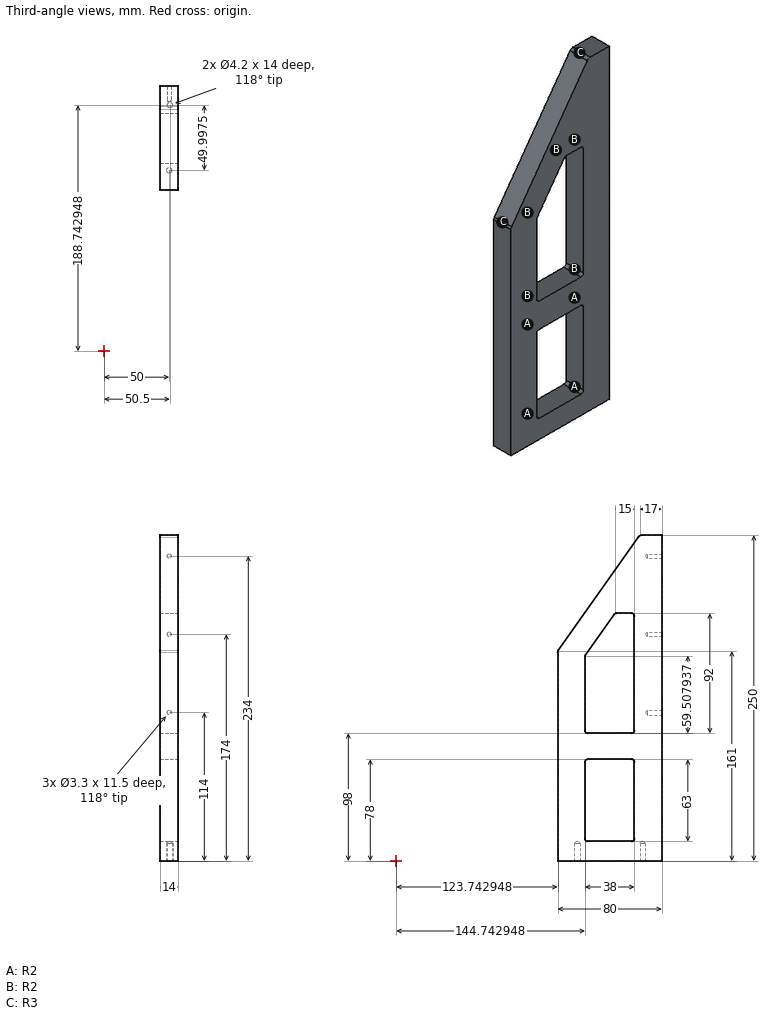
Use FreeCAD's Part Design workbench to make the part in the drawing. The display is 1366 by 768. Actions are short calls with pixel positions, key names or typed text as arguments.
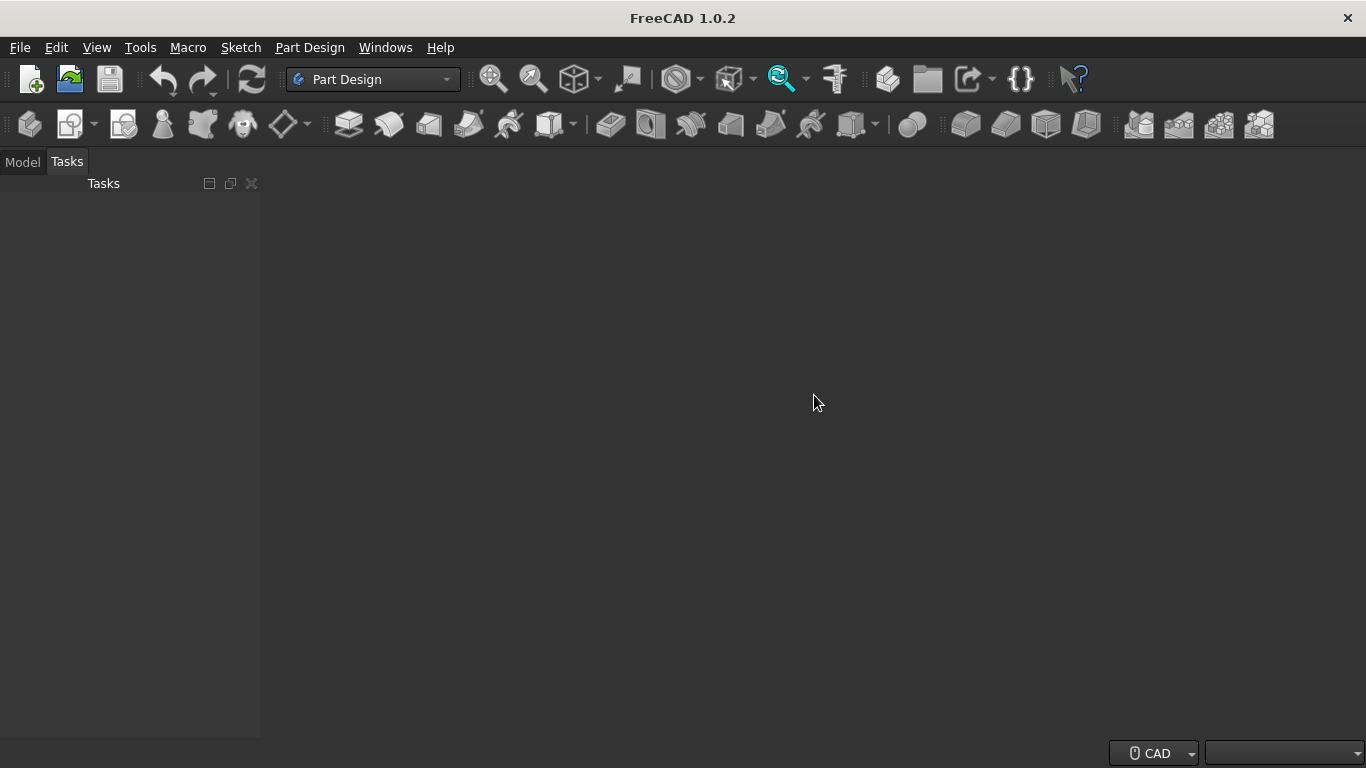
click(30, 80)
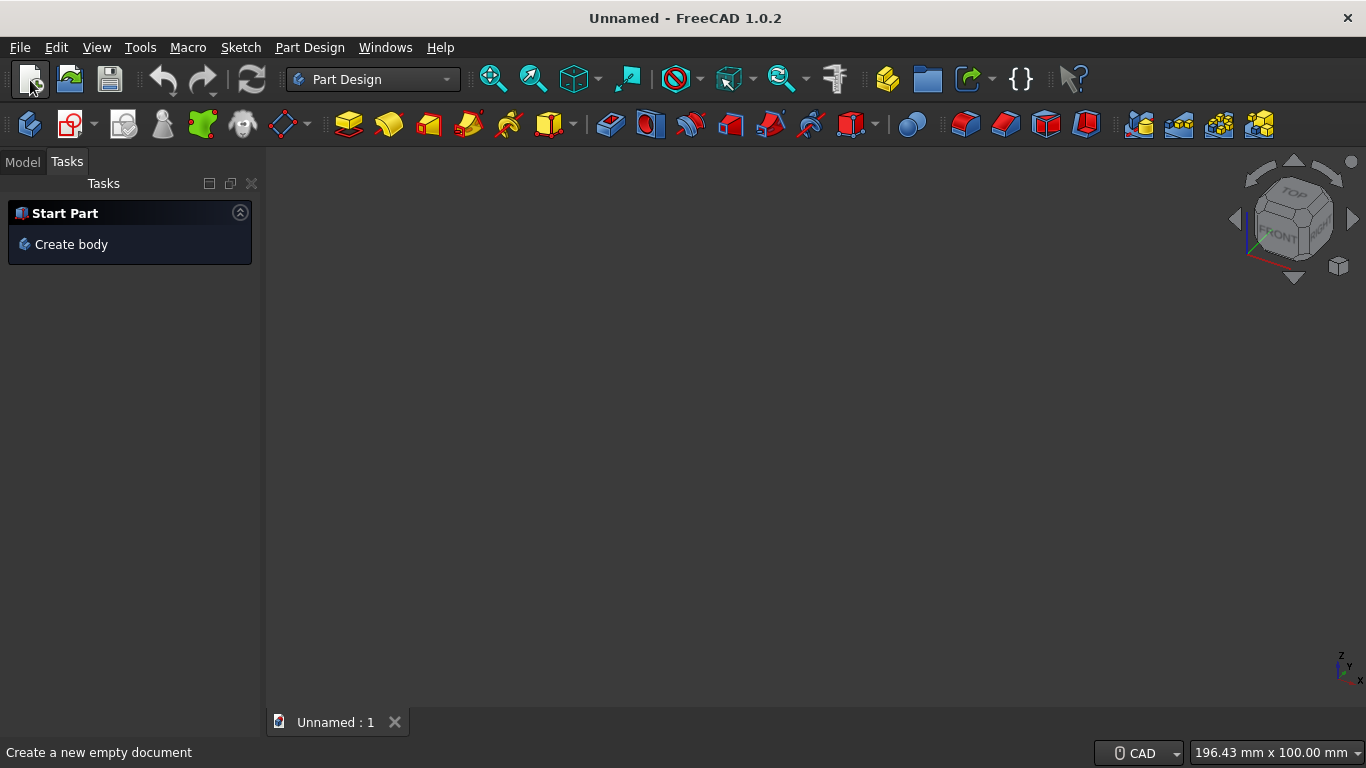
click(30, 124)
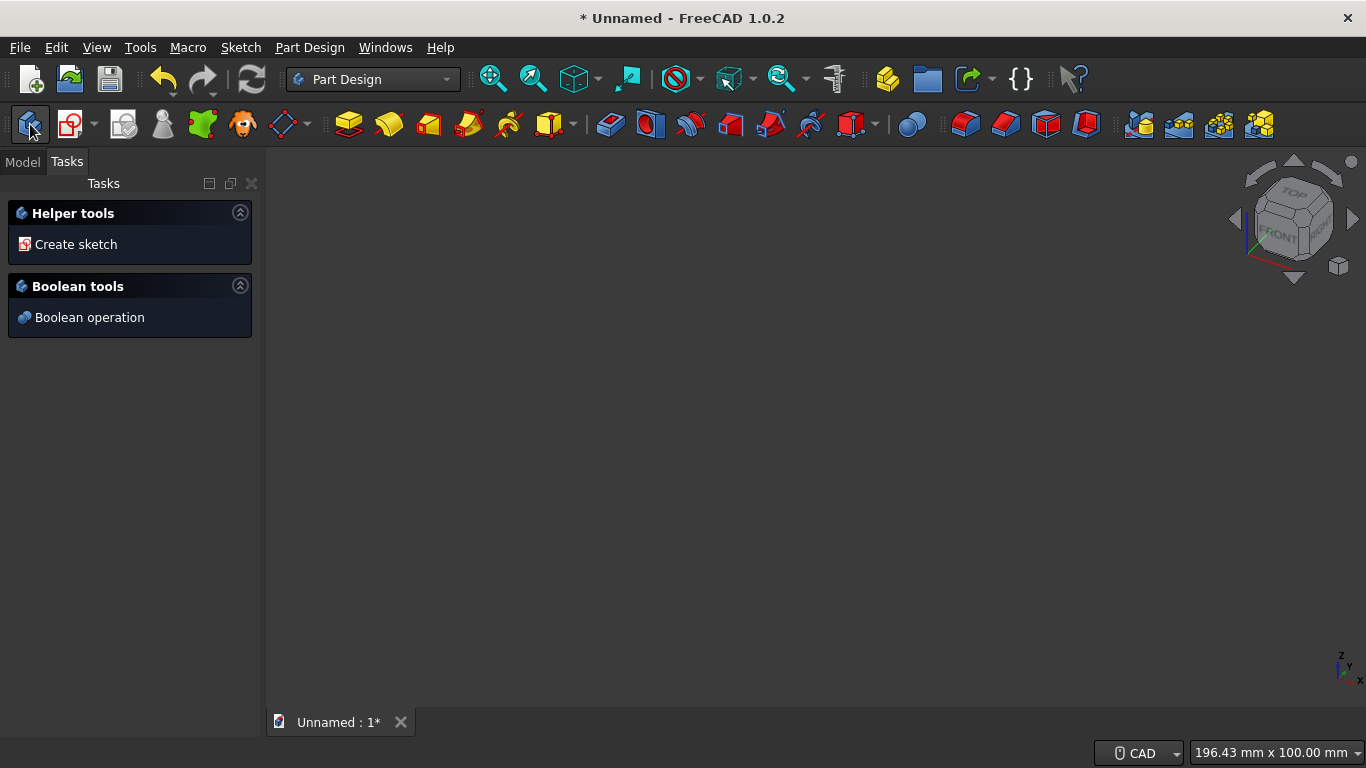
click(23, 161)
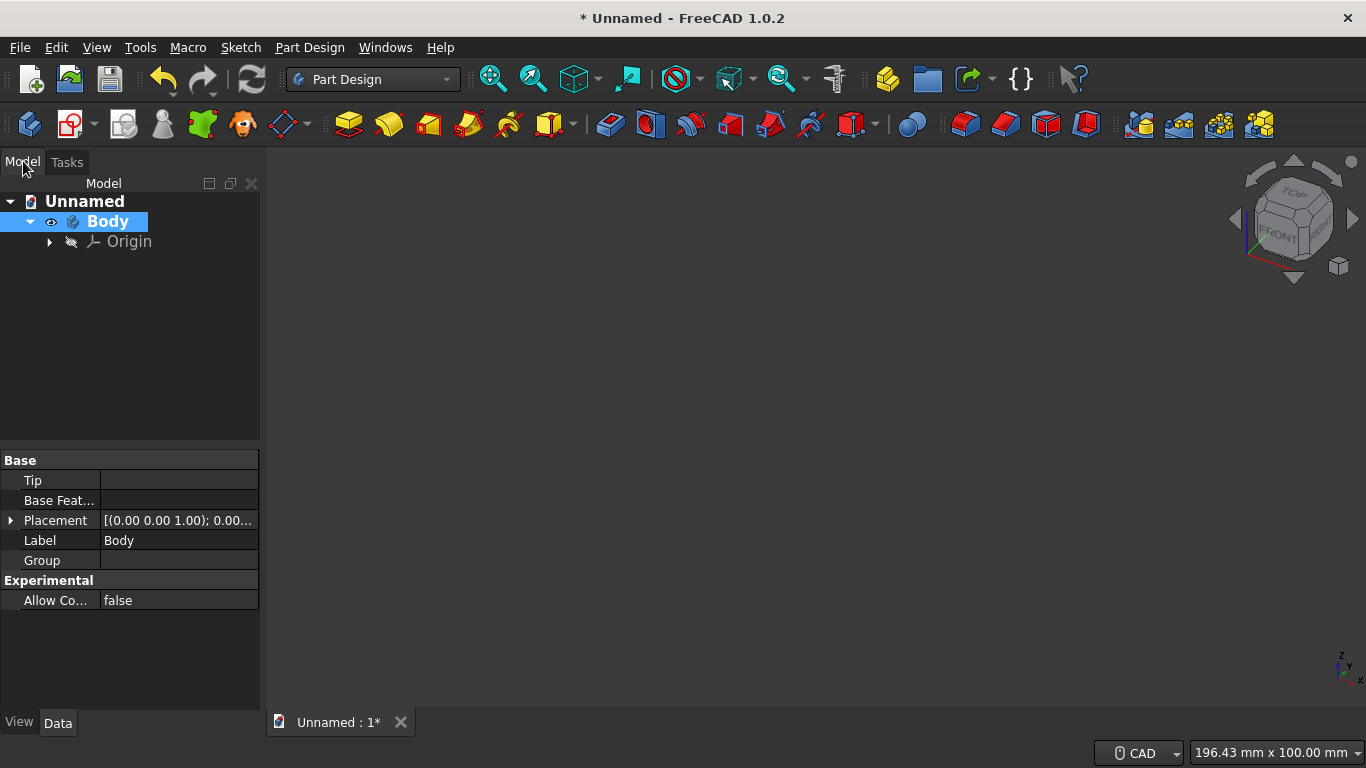
click(50, 242)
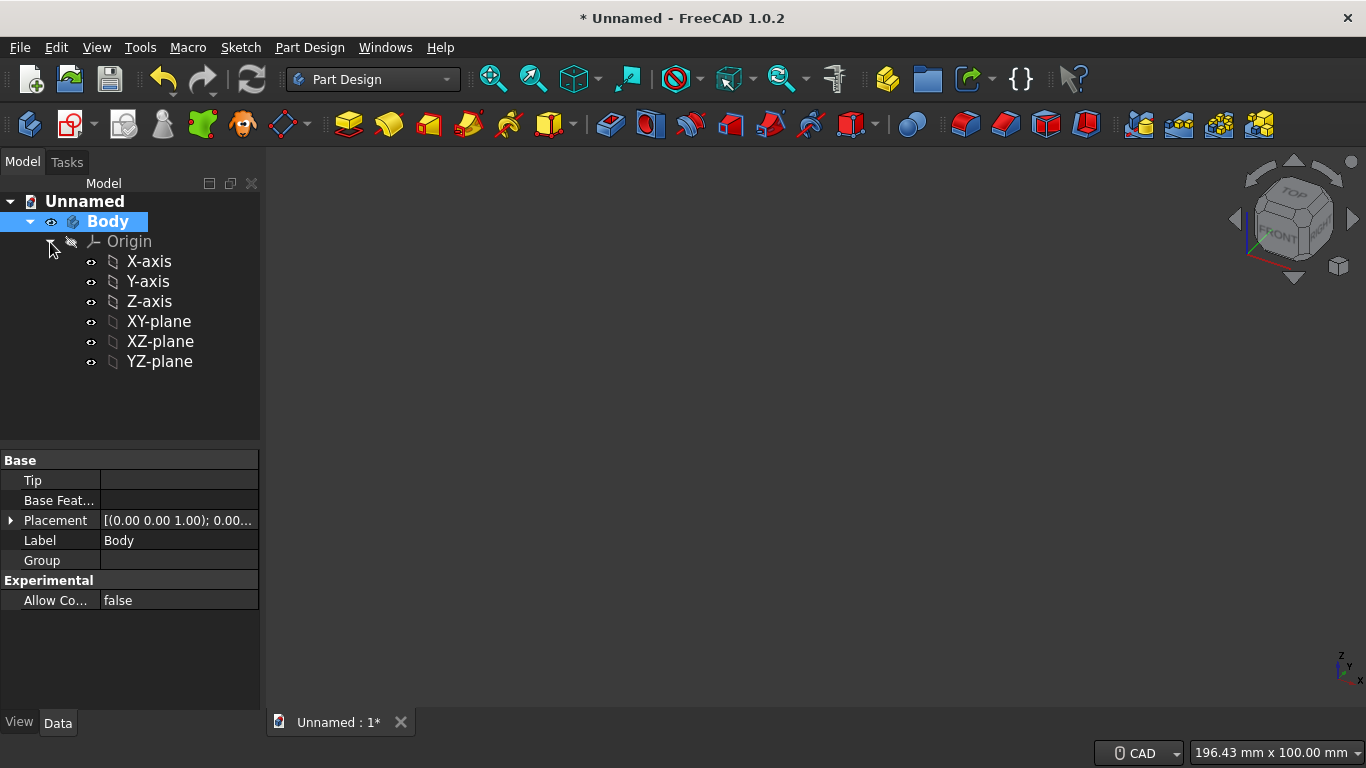
click(136, 362)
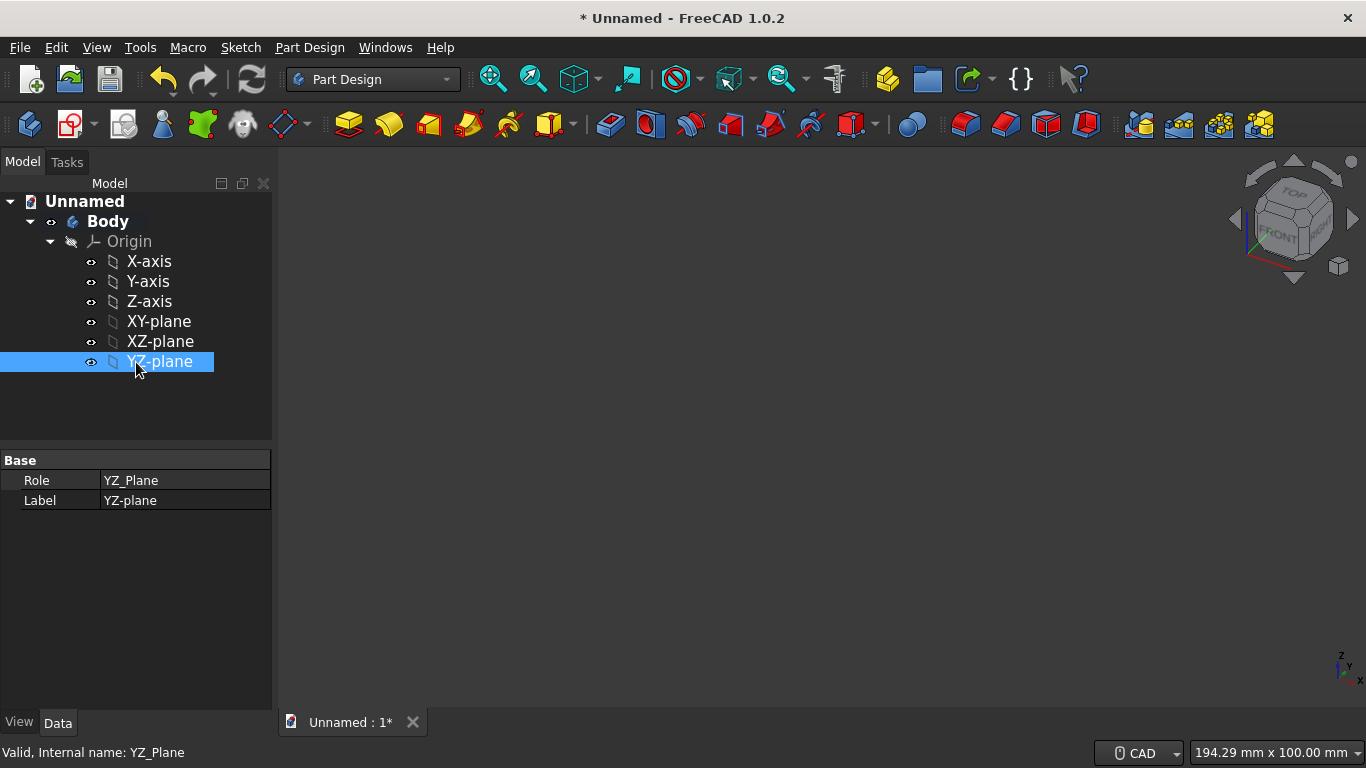
click(284, 124)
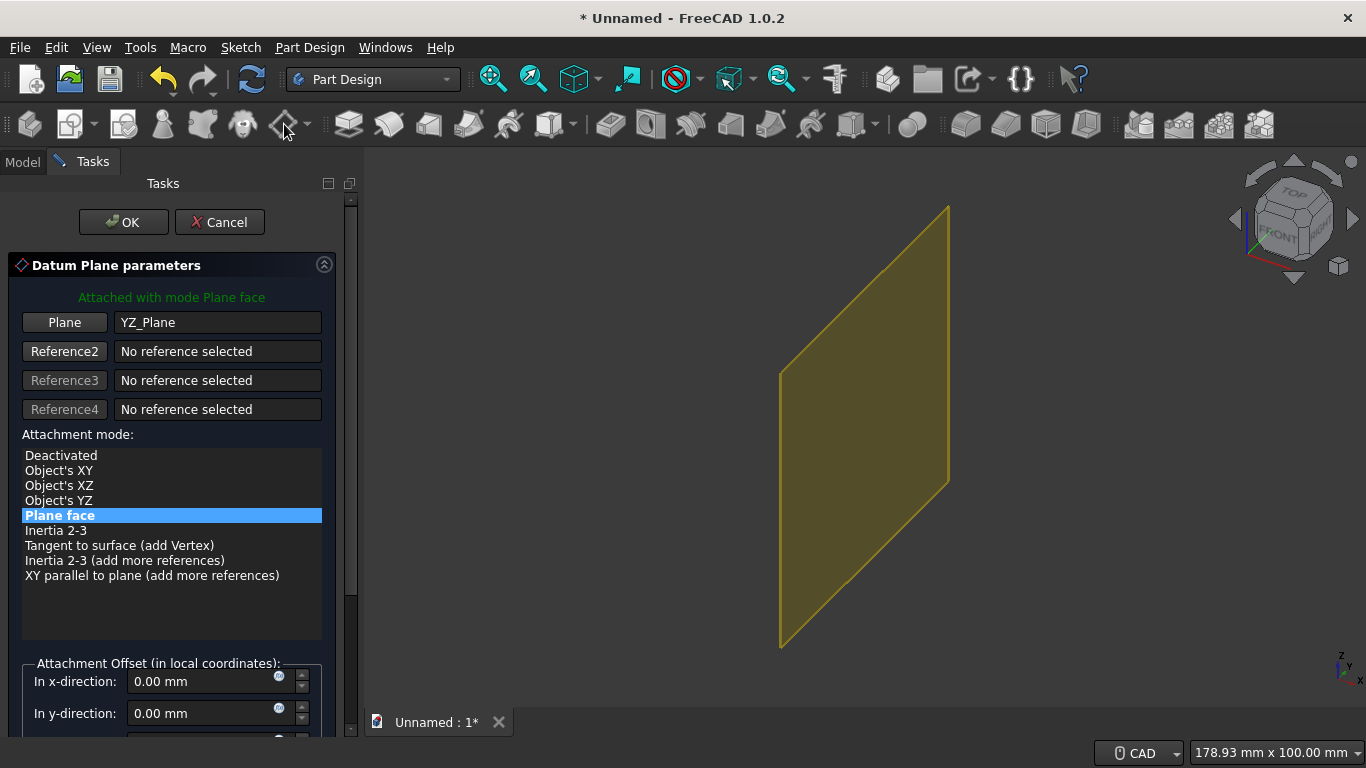
scroll(351, 464, down, 2)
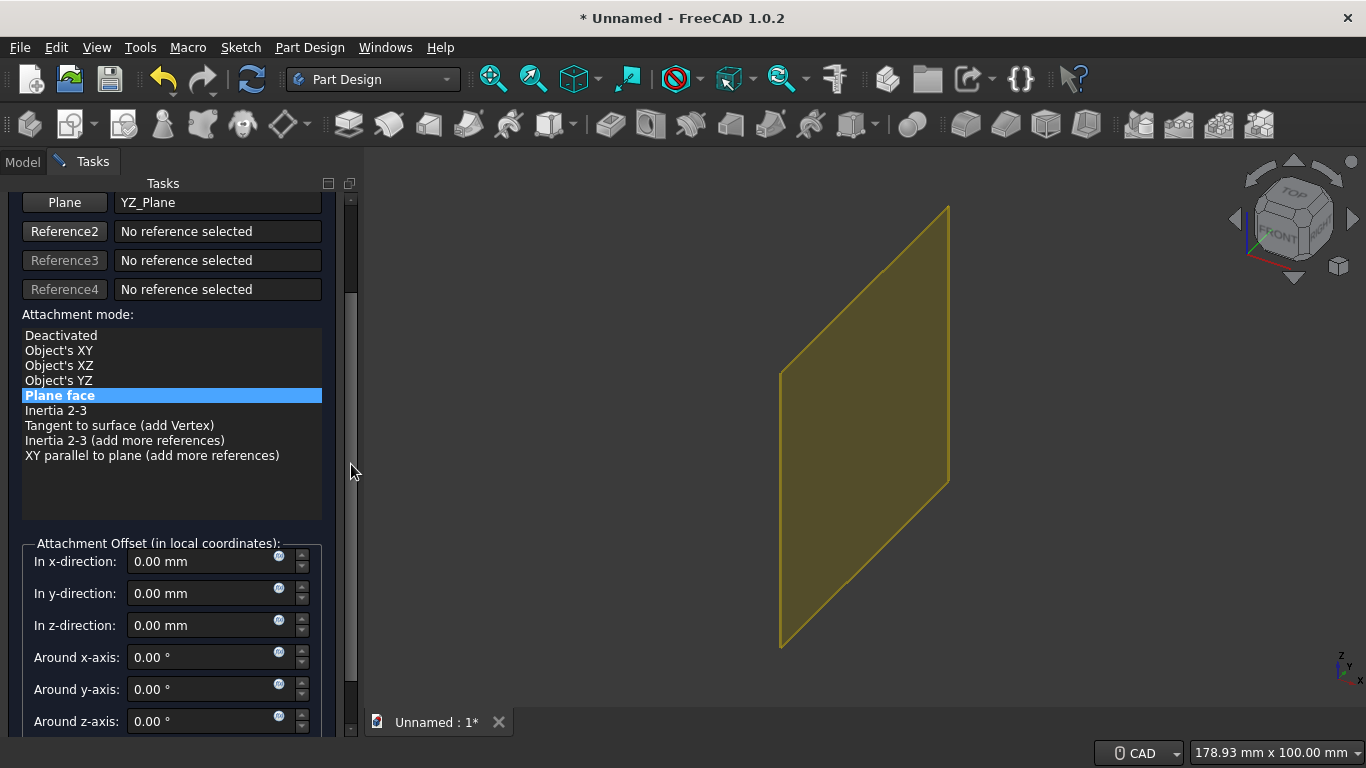
triple_click(210, 625)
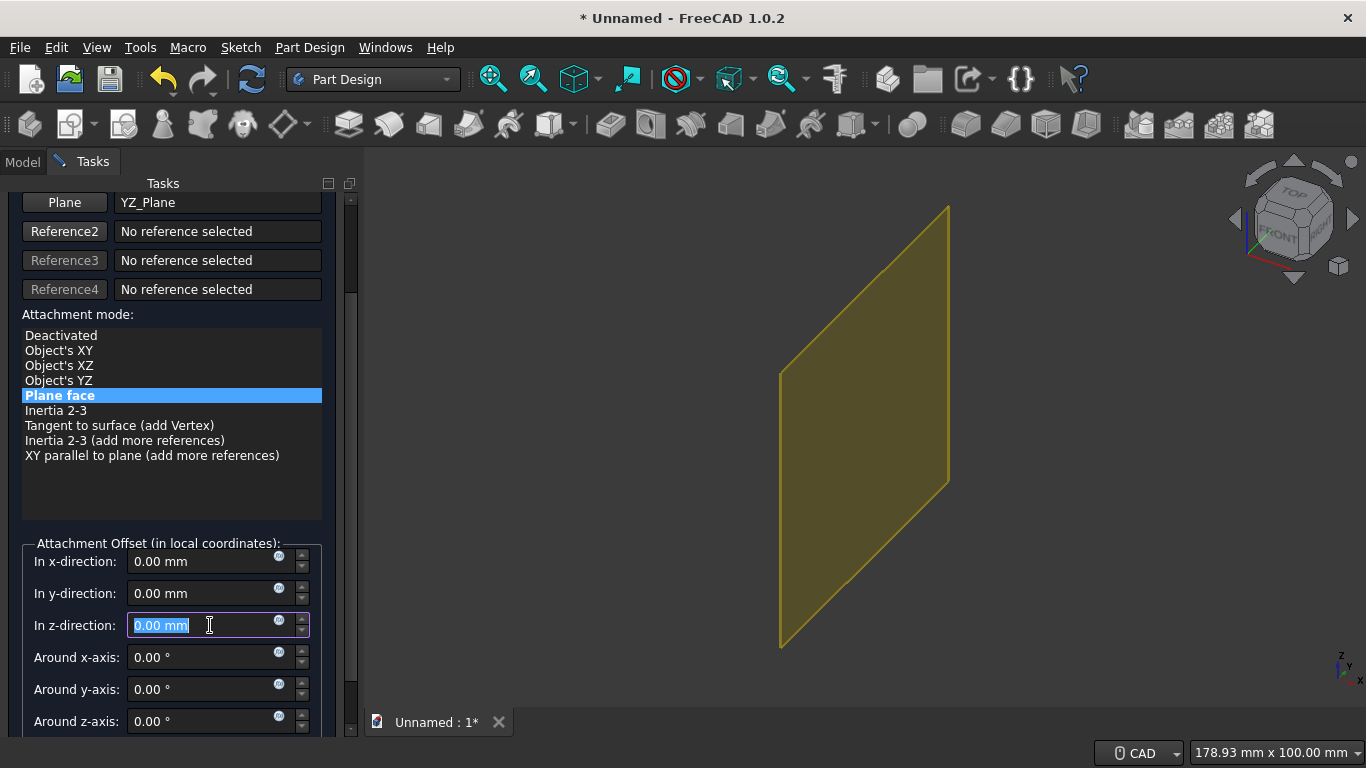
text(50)
key(Tab)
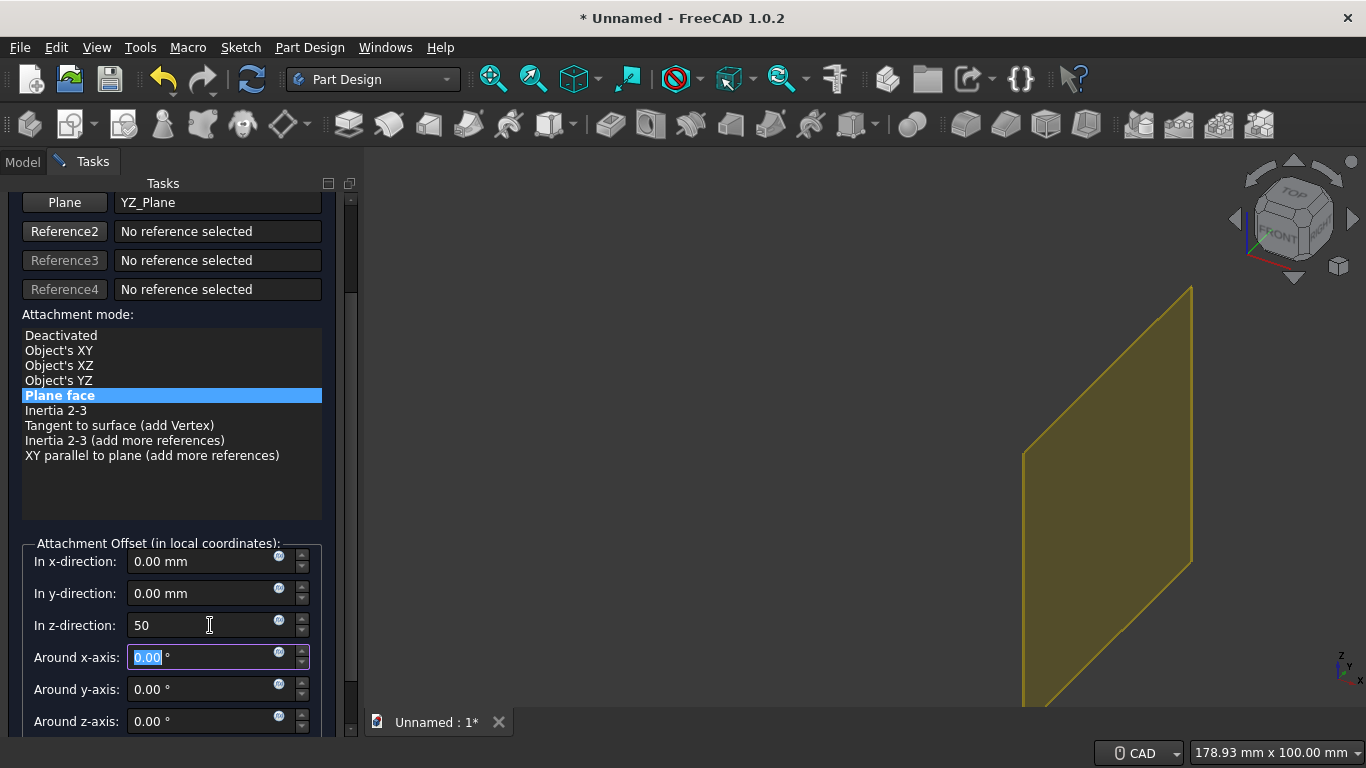
scroll(351, 464, up, 3)